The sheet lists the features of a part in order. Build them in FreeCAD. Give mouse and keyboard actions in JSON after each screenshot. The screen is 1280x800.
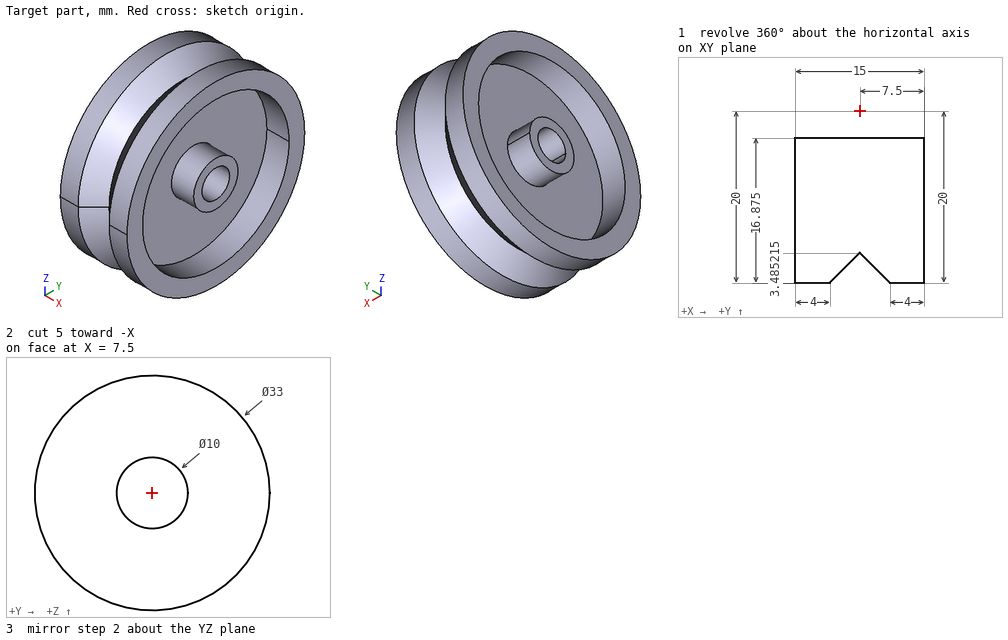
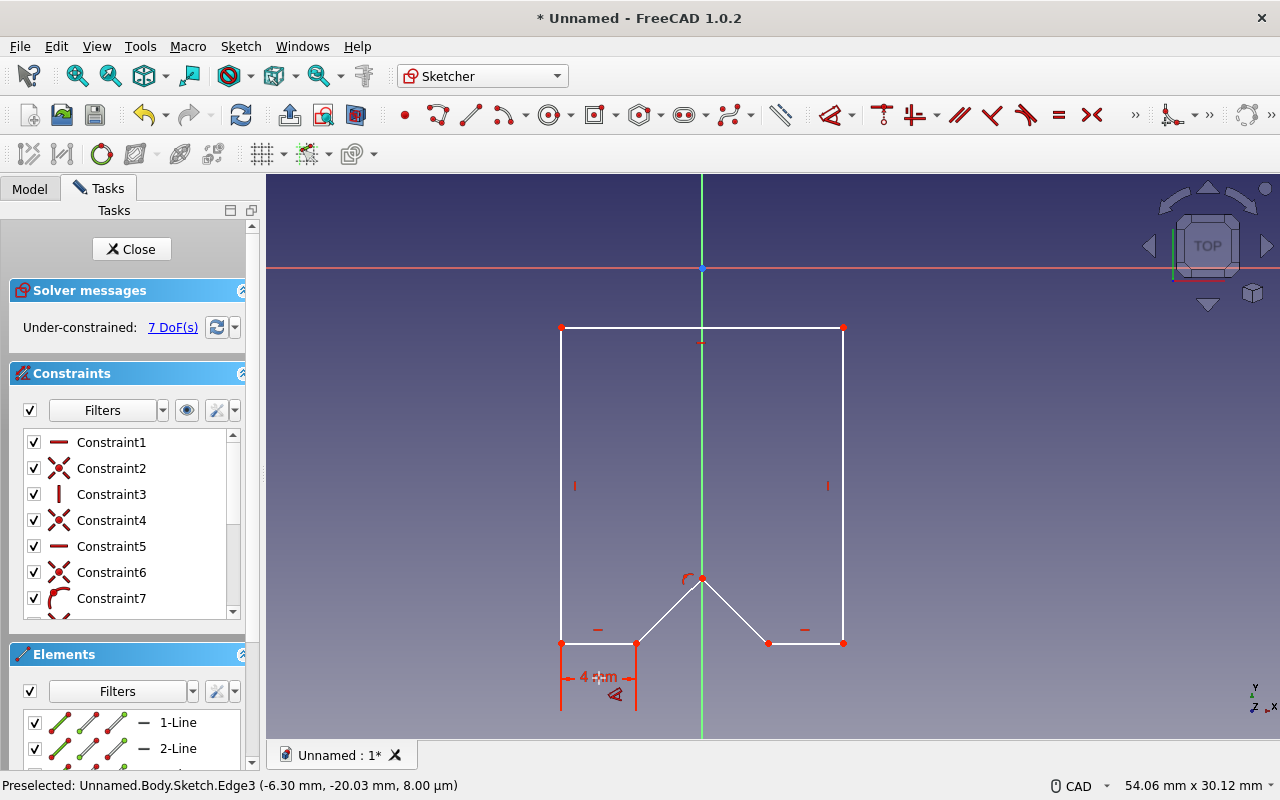
{"action": "left_click", "coordinate": [790, 644]}
{"action": "left_click", "coordinate": [805, 678]}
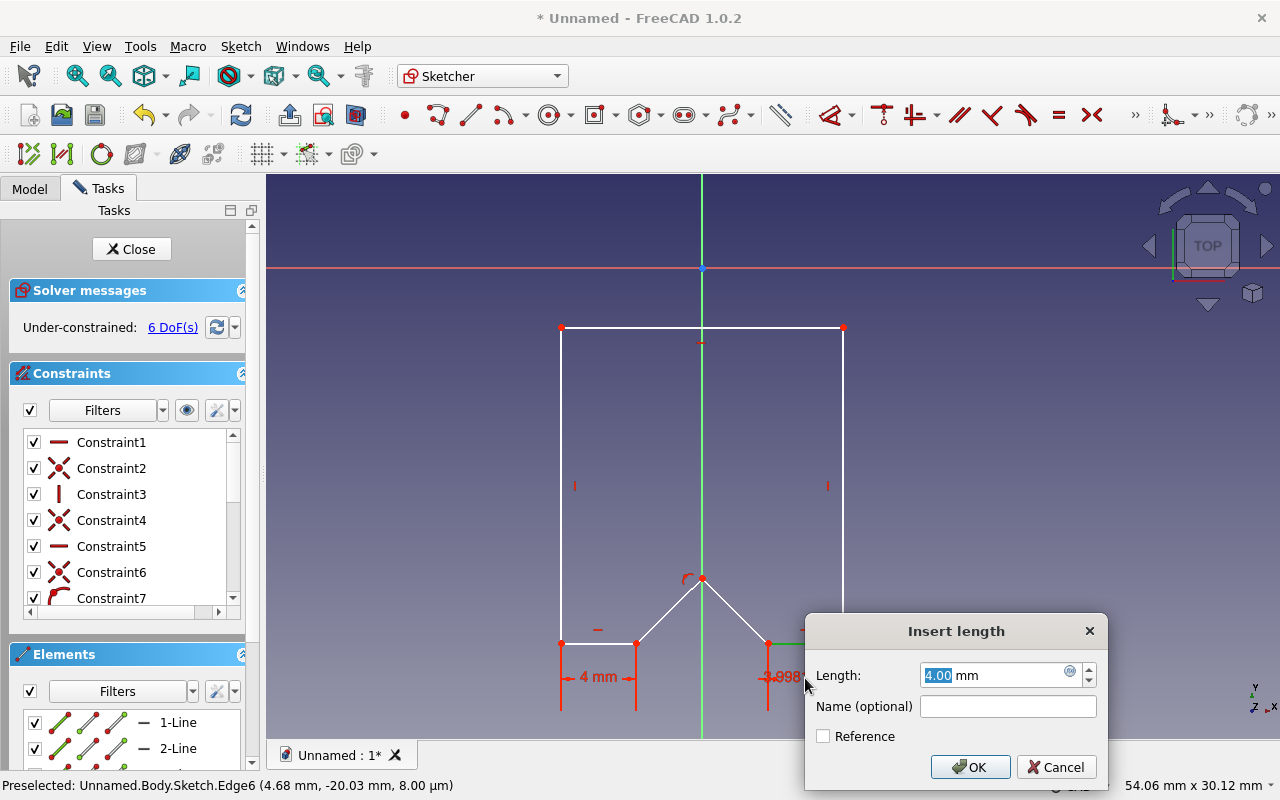
{"action": "type", "text": "4"}
{"action": "key", "text": "Return"}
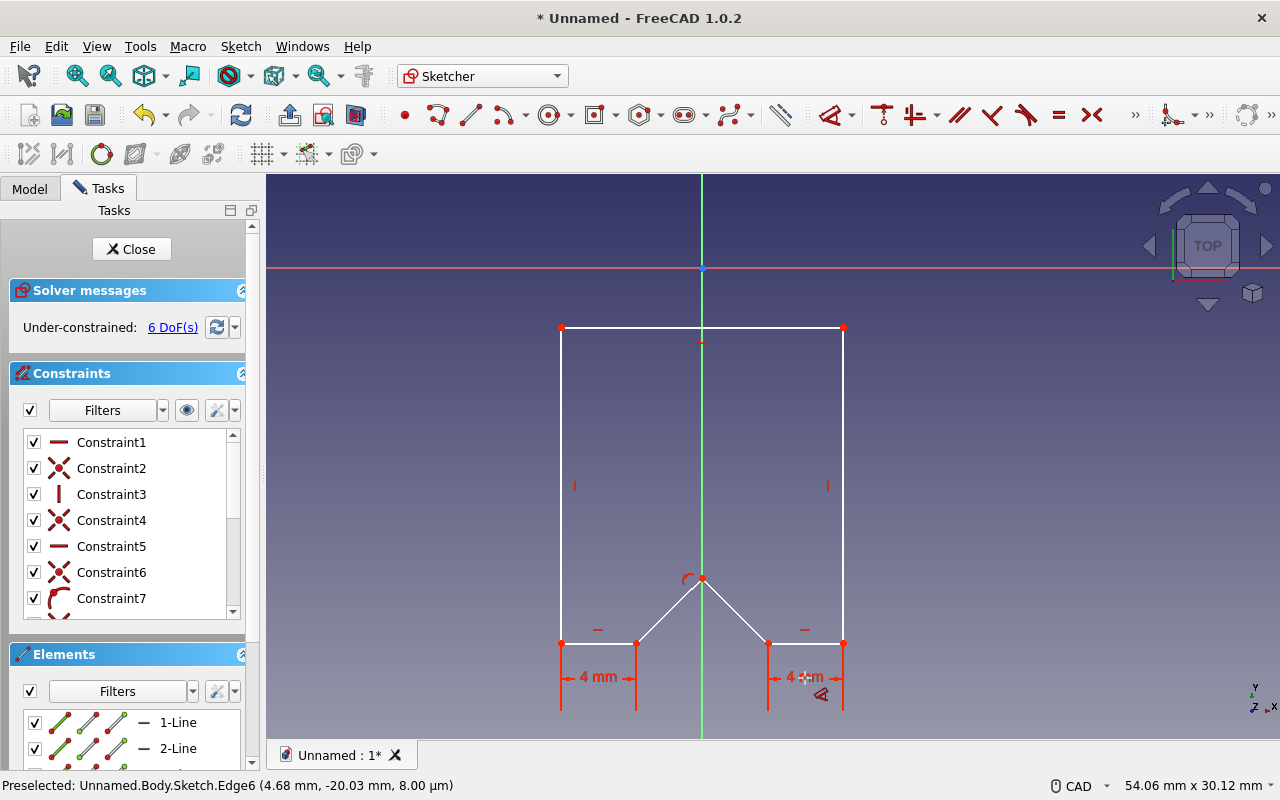
{"action": "left_click", "coordinate": [758, 328]}
{"action": "left_click", "coordinate": [637, 294]}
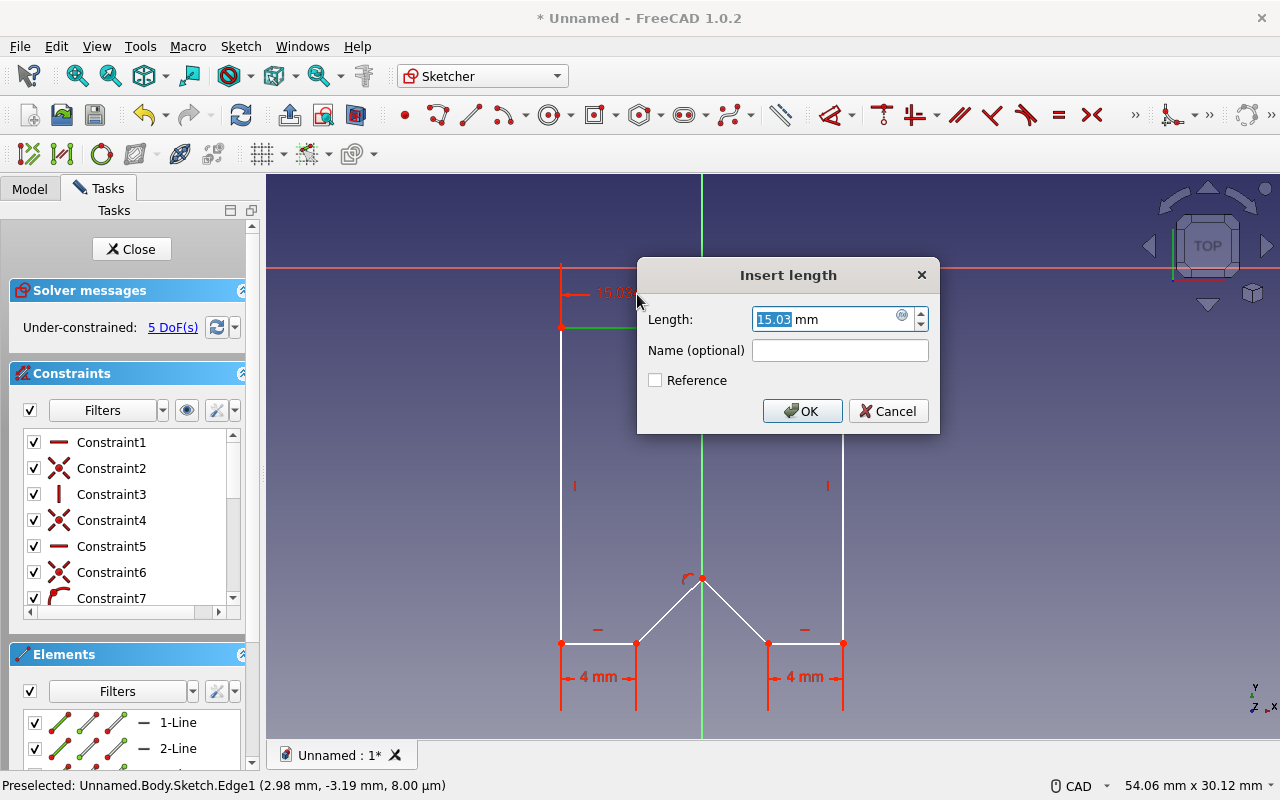
{"action": "type", "text": "15"}
{"action": "key", "text": "Return"}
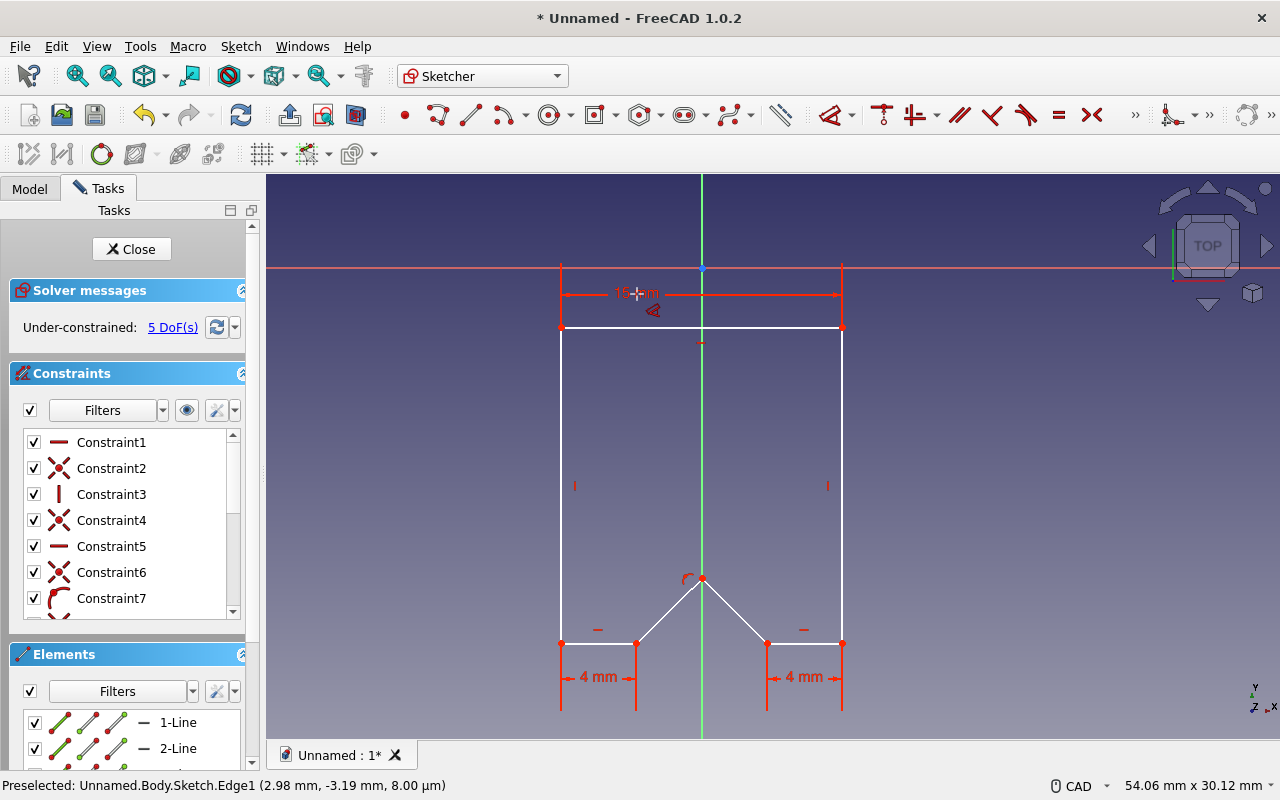
{"action": "left_click", "coordinate": [561, 644]}
{"action": "left_click", "coordinate": [527, 456]}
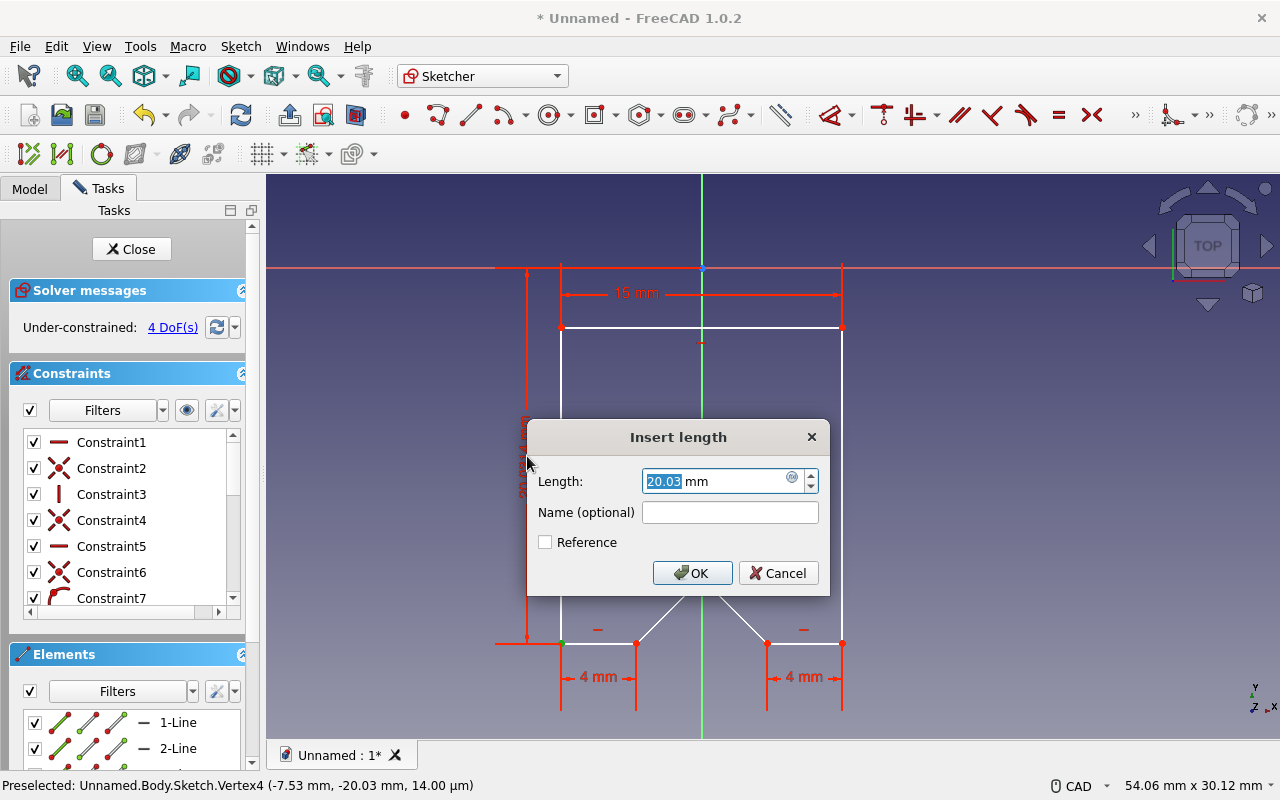
{"action": "type", "text": "20"}
{"action": "key", "text": "Return"}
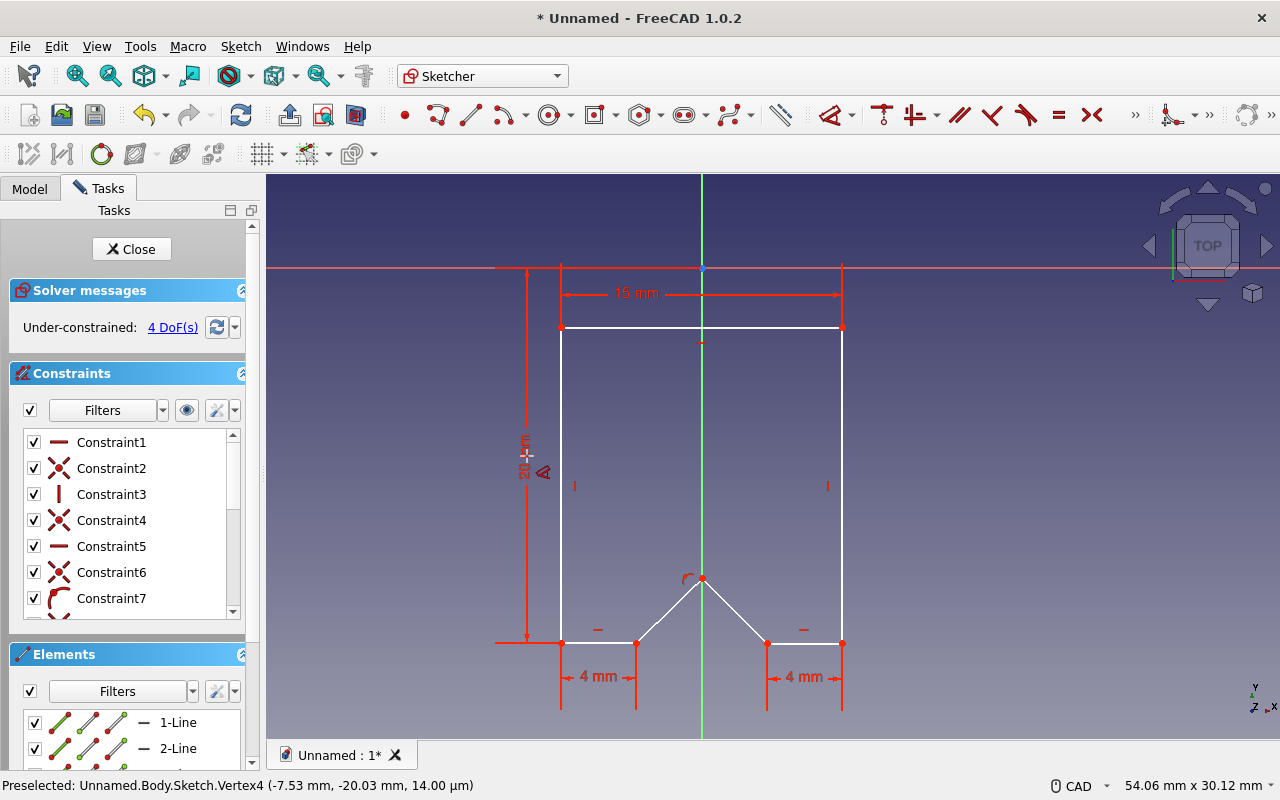
{"action": "left_click", "coordinate": [767, 644]}
{"action": "left_click", "coordinate": [801, 456]}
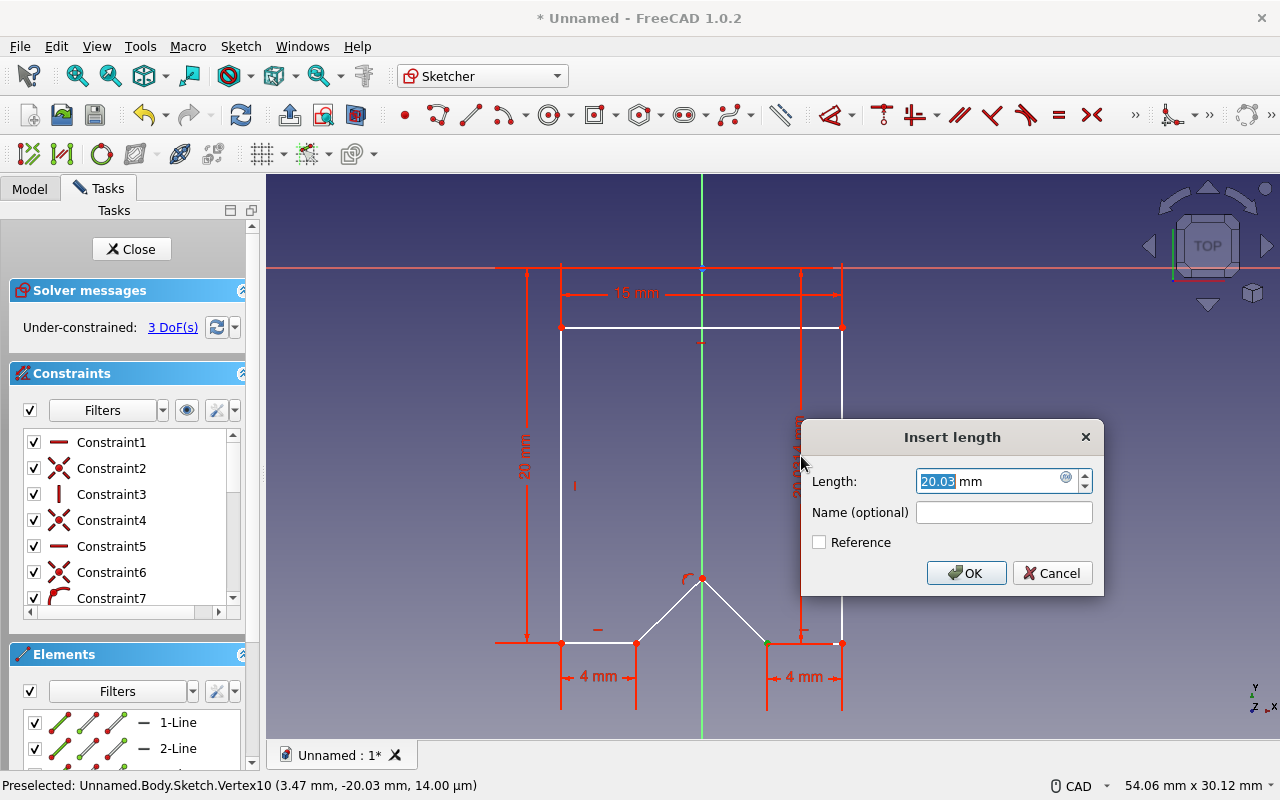
{"action": "type", "text": "20"}
{"action": "key", "text": "Return"}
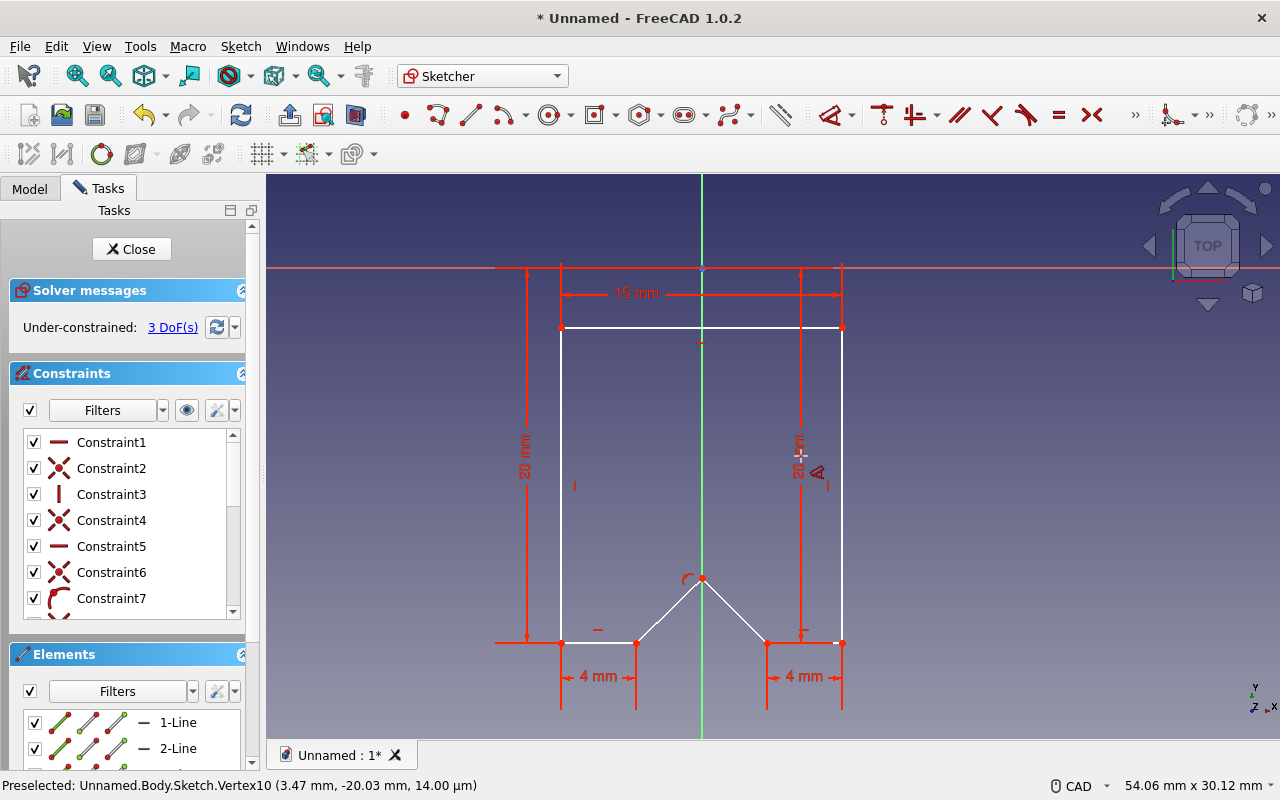
{"action": "left_click", "coordinate": [842, 328]}
{"action": "left_click", "coordinate": [772, 234]}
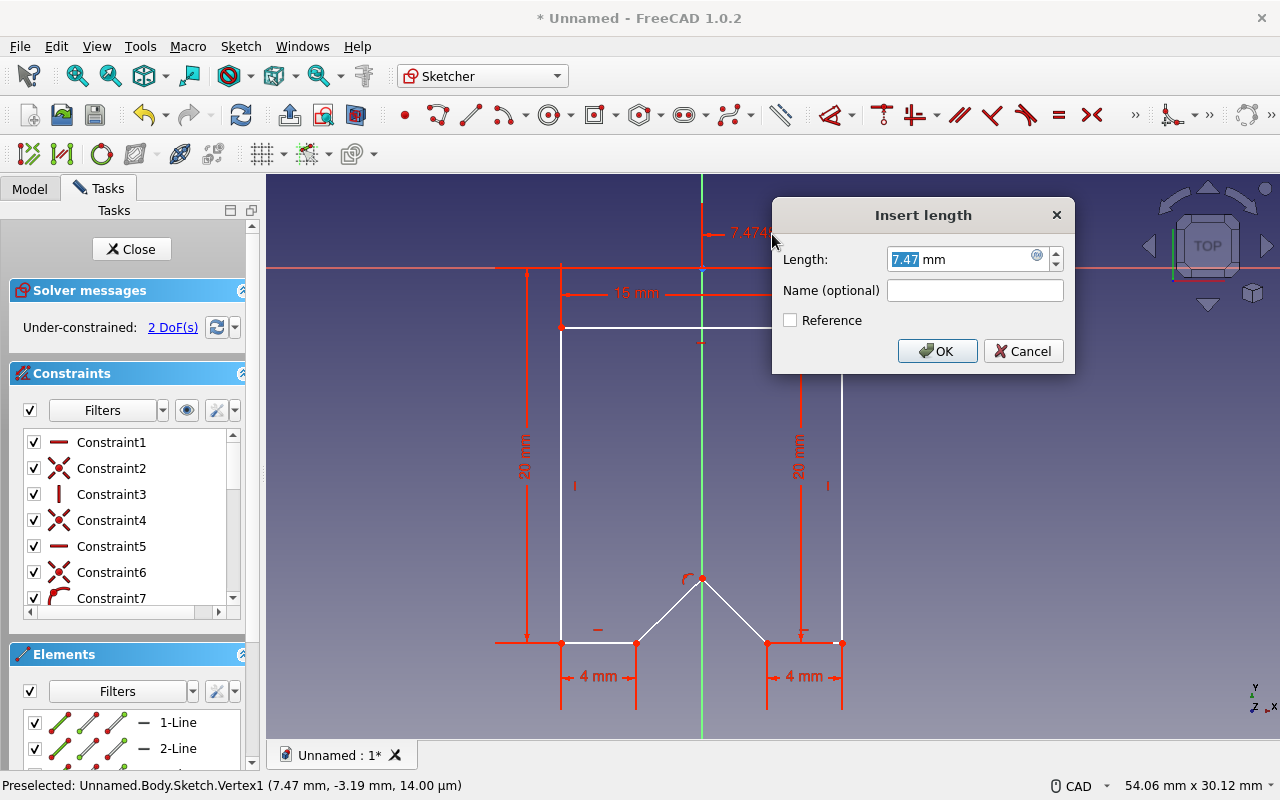
{"action": "type", "text": "7.5"}
{"action": "key", "text": "Return"}